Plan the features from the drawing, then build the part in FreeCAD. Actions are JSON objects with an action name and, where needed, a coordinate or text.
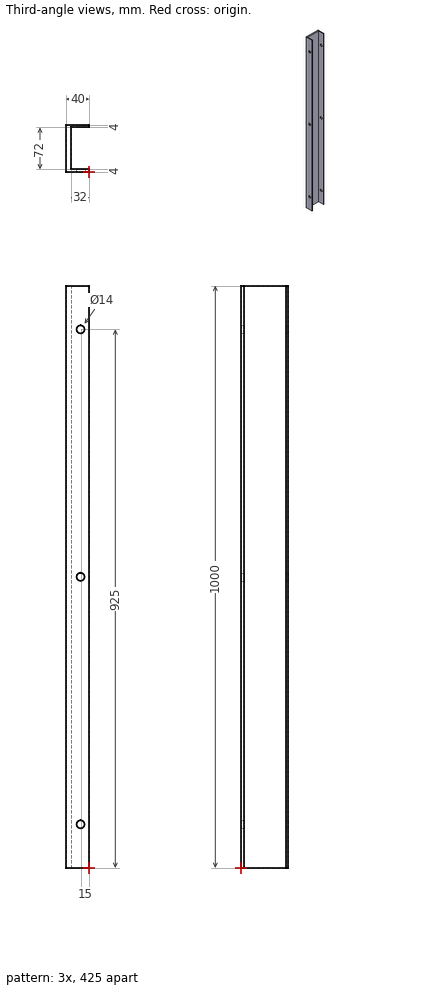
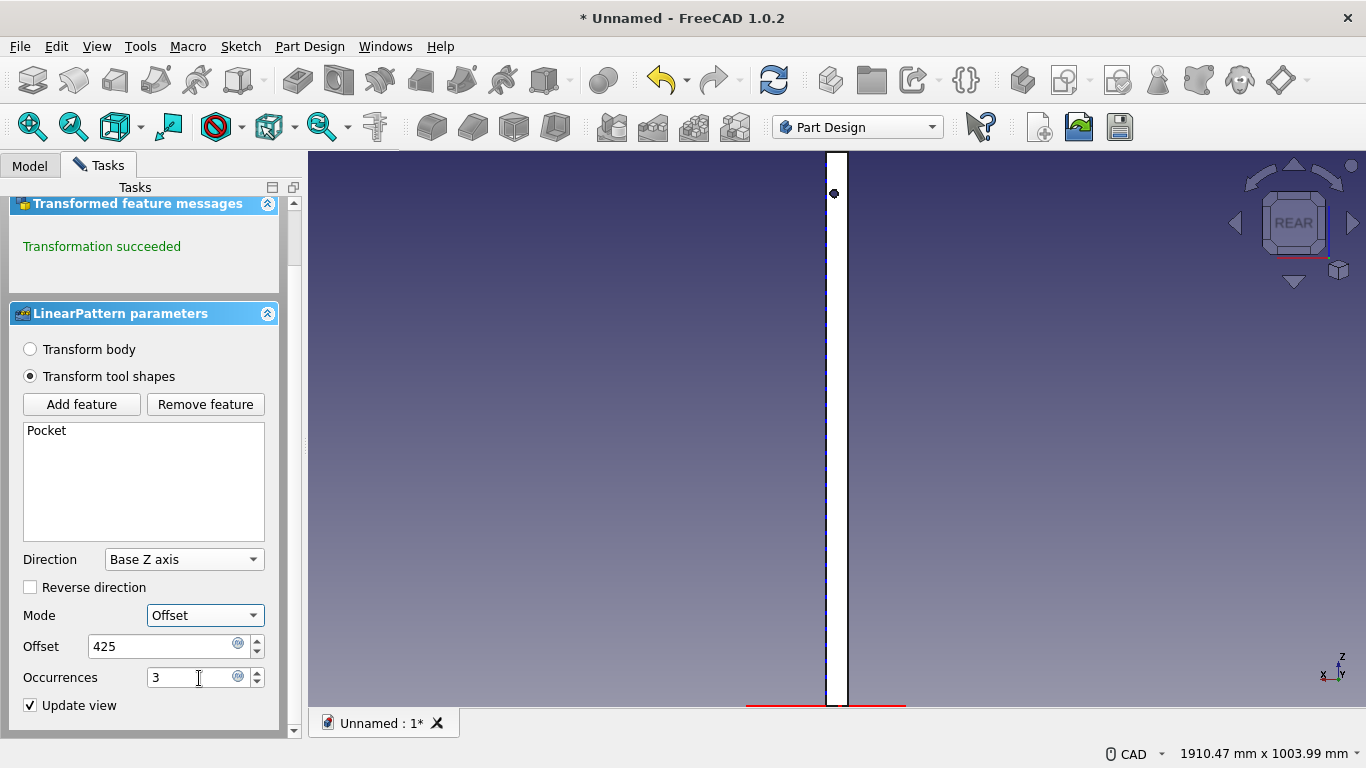
{"action": "left_click", "coordinate": [31, 587]}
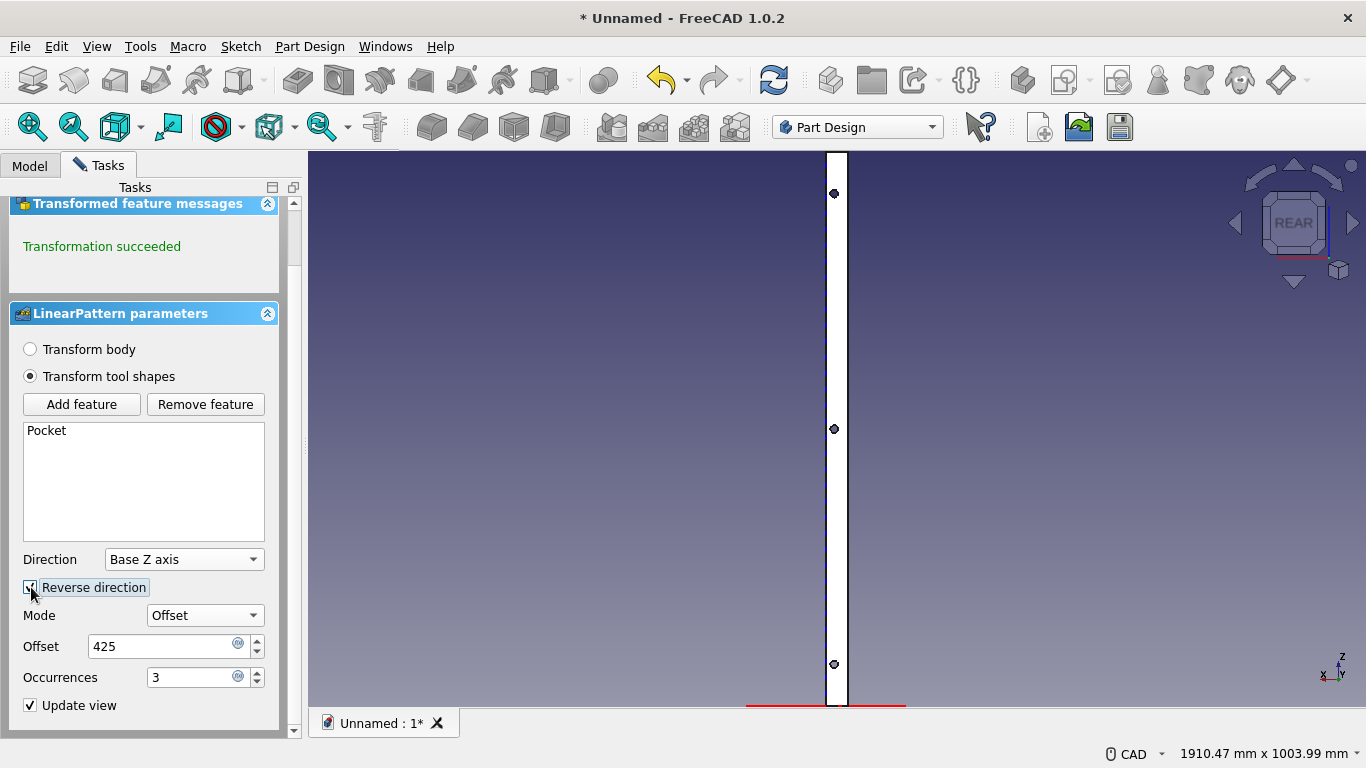
{"action": "scroll", "coordinate": [294, 468], "scroll_direction": "up", "scroll_amount": 2}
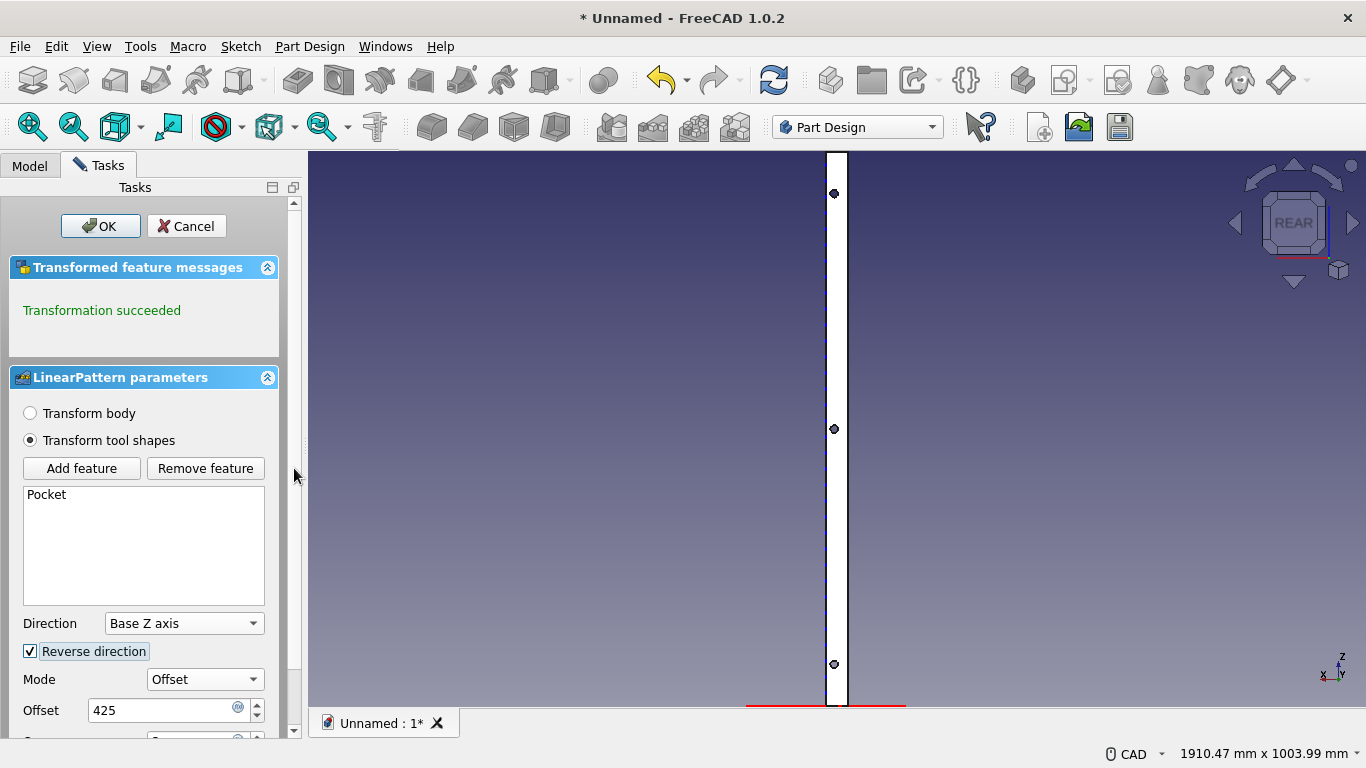
{"action": "left_click", "coordinate": [101, 226]}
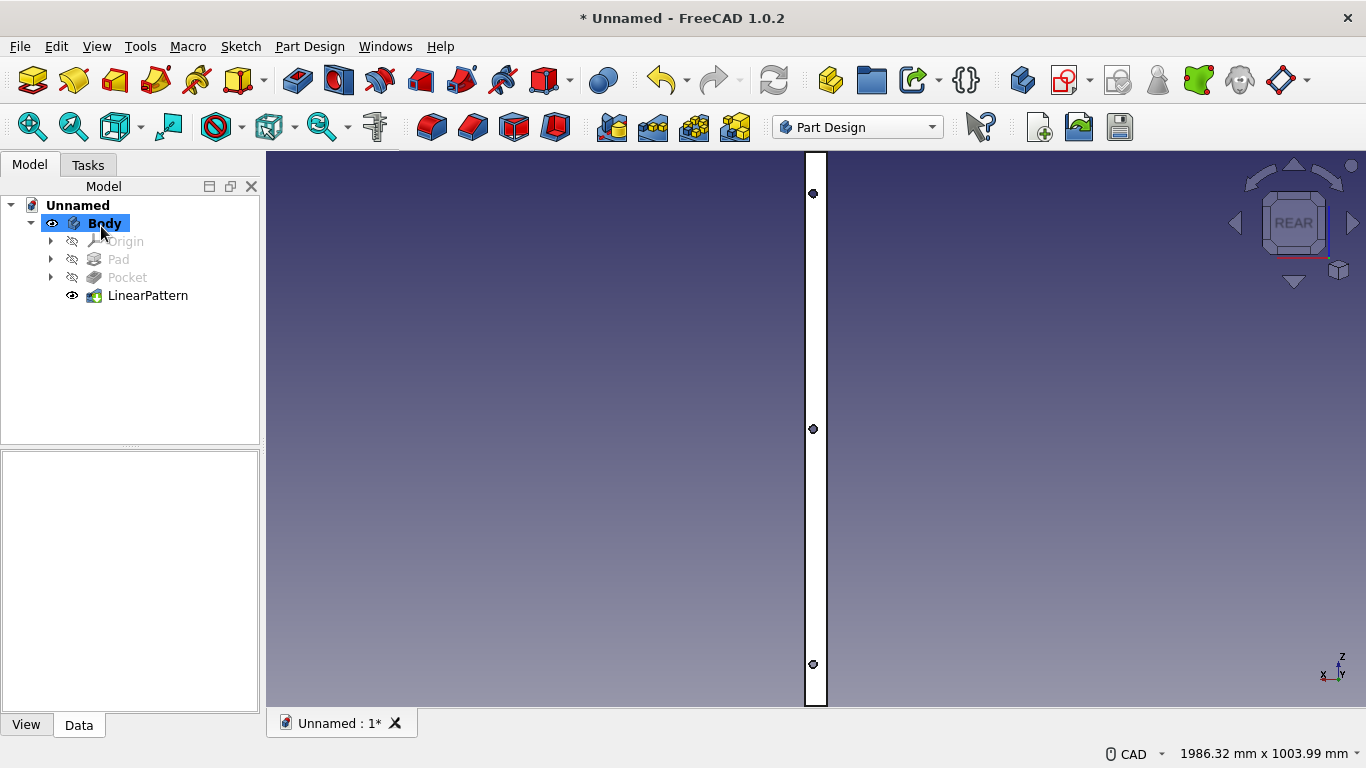
{"action": "key", "text": "0"}